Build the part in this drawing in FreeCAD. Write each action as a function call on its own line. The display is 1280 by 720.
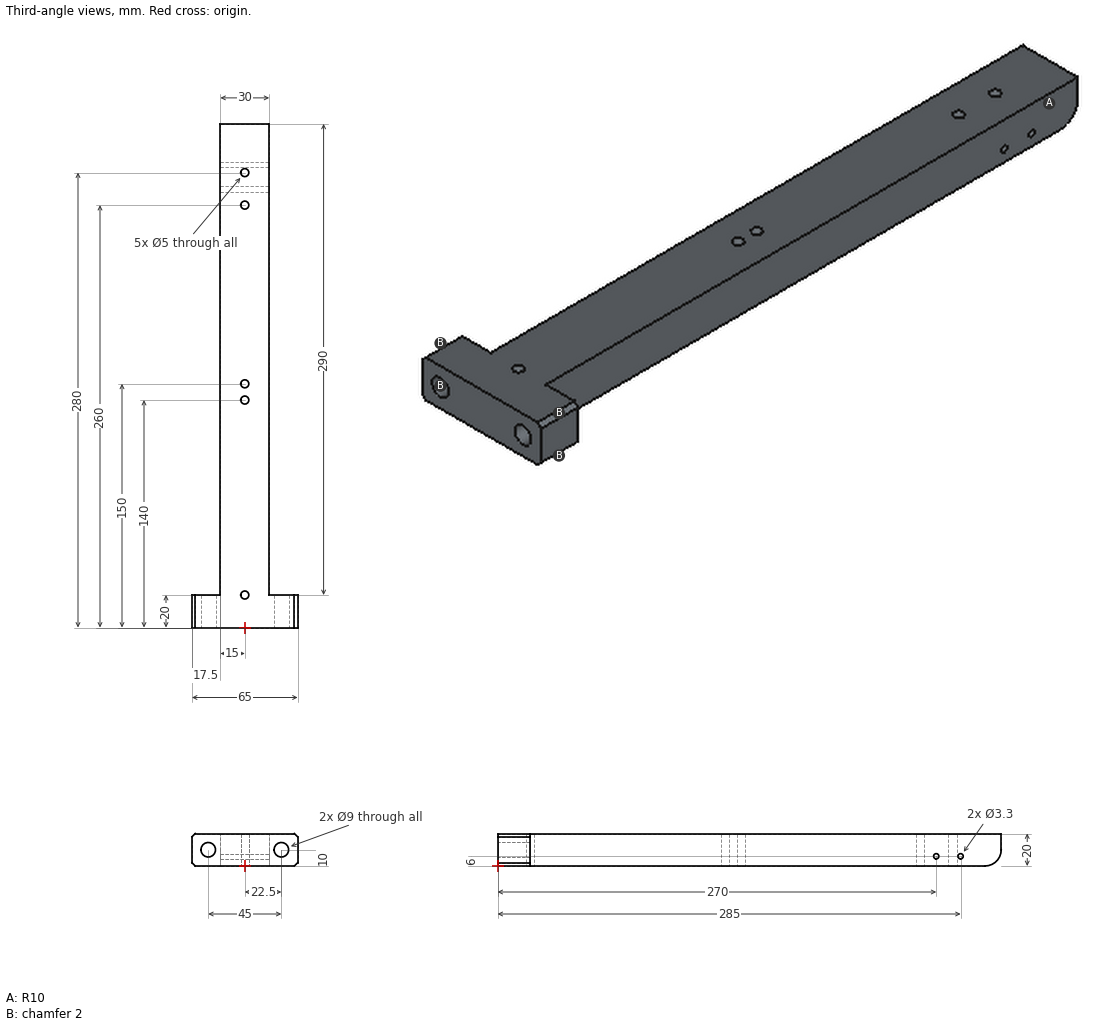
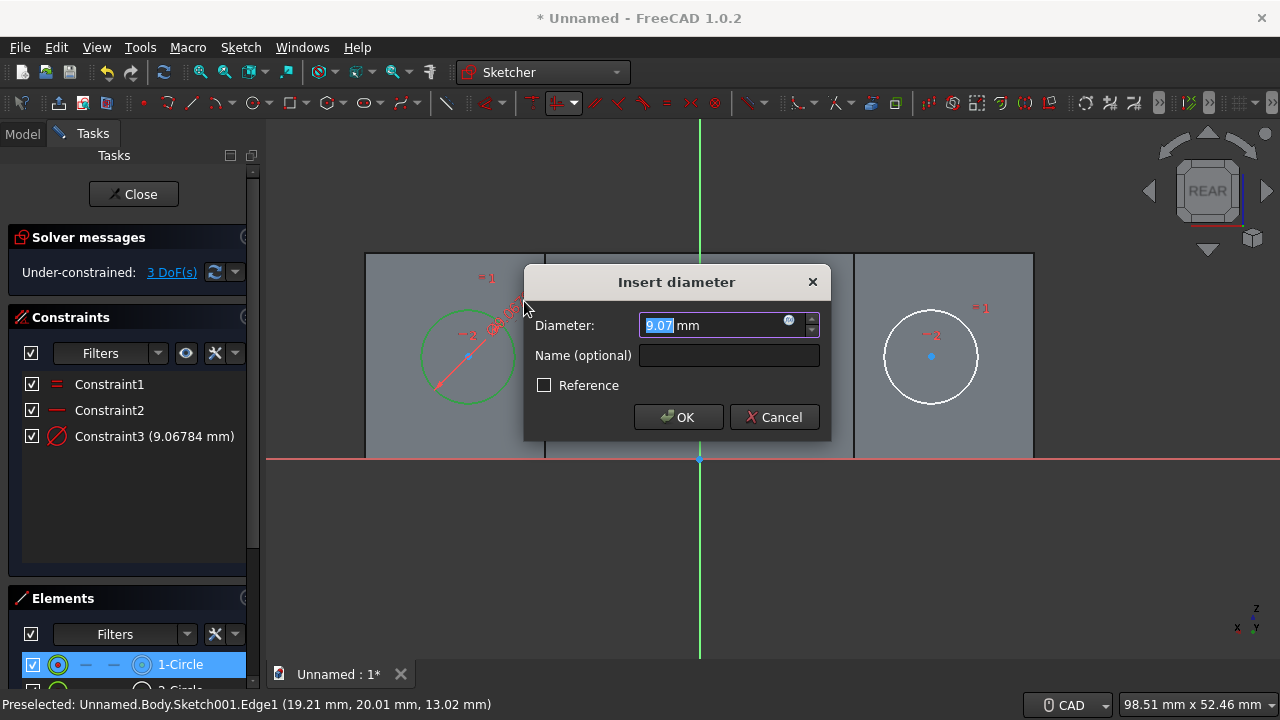
text(9)
key(Return)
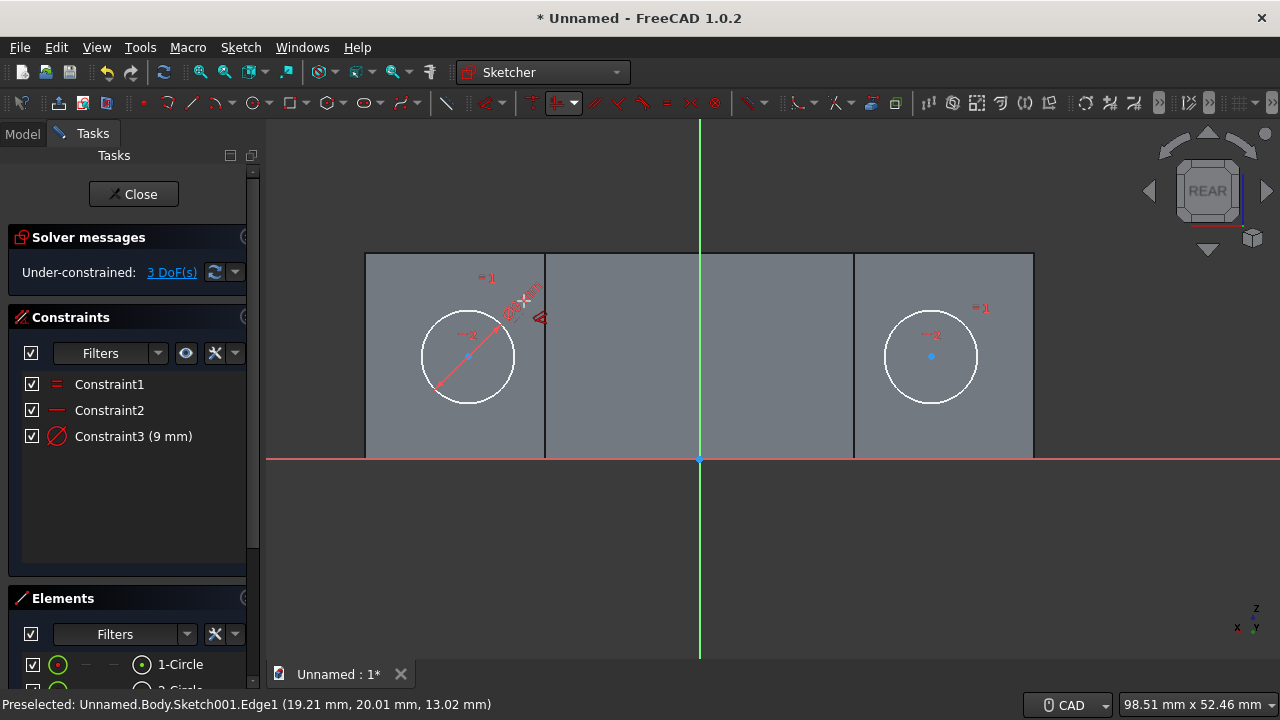
click(468, 357)
click(434, 408)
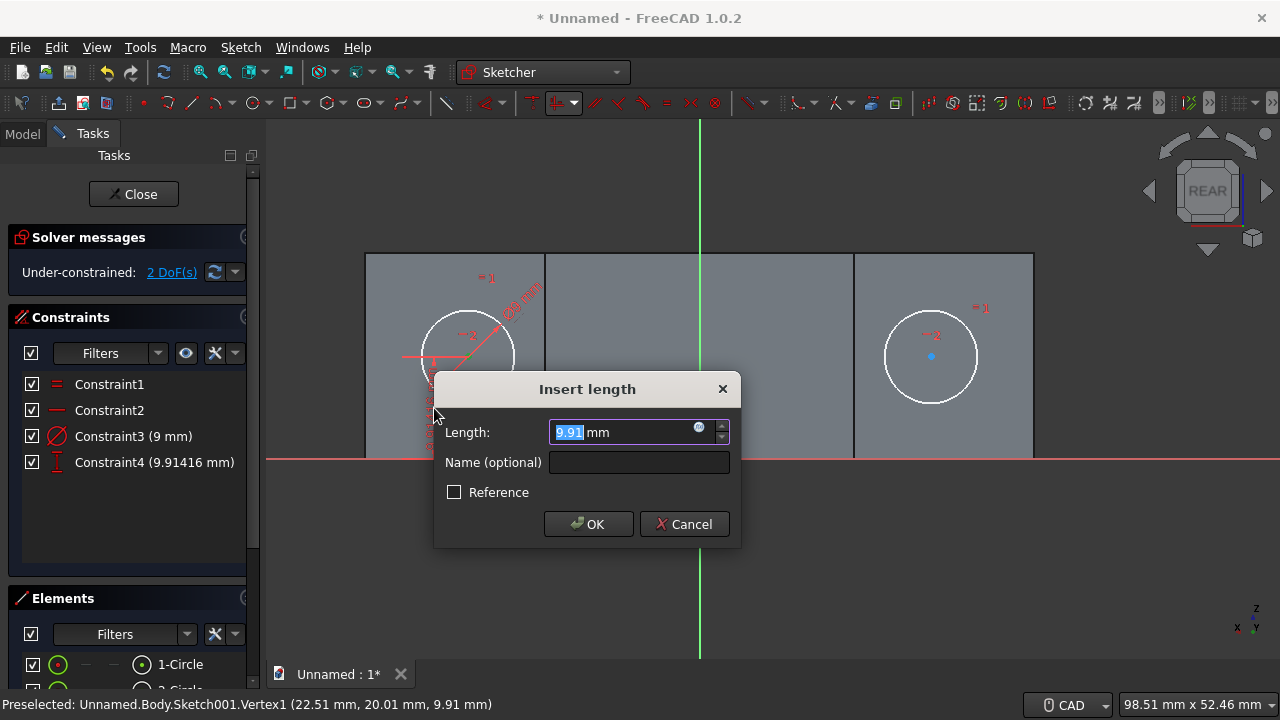
text(10)
key(Return)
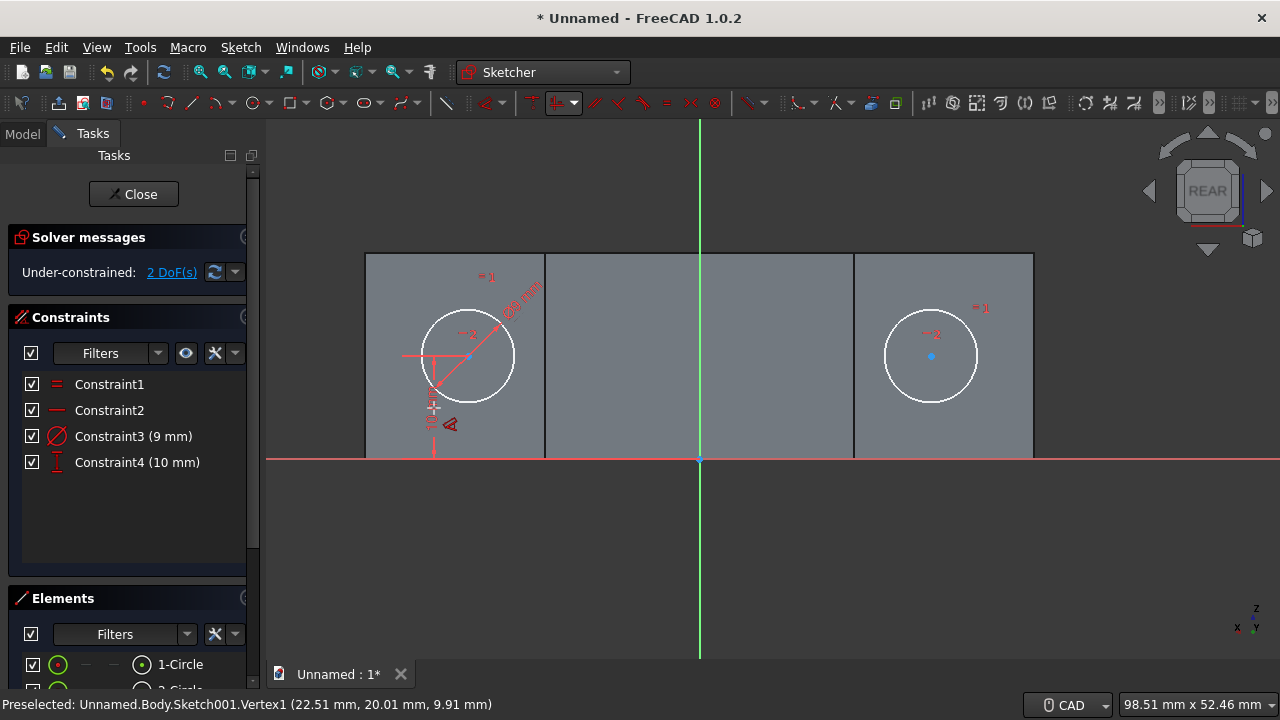
click(468, 356)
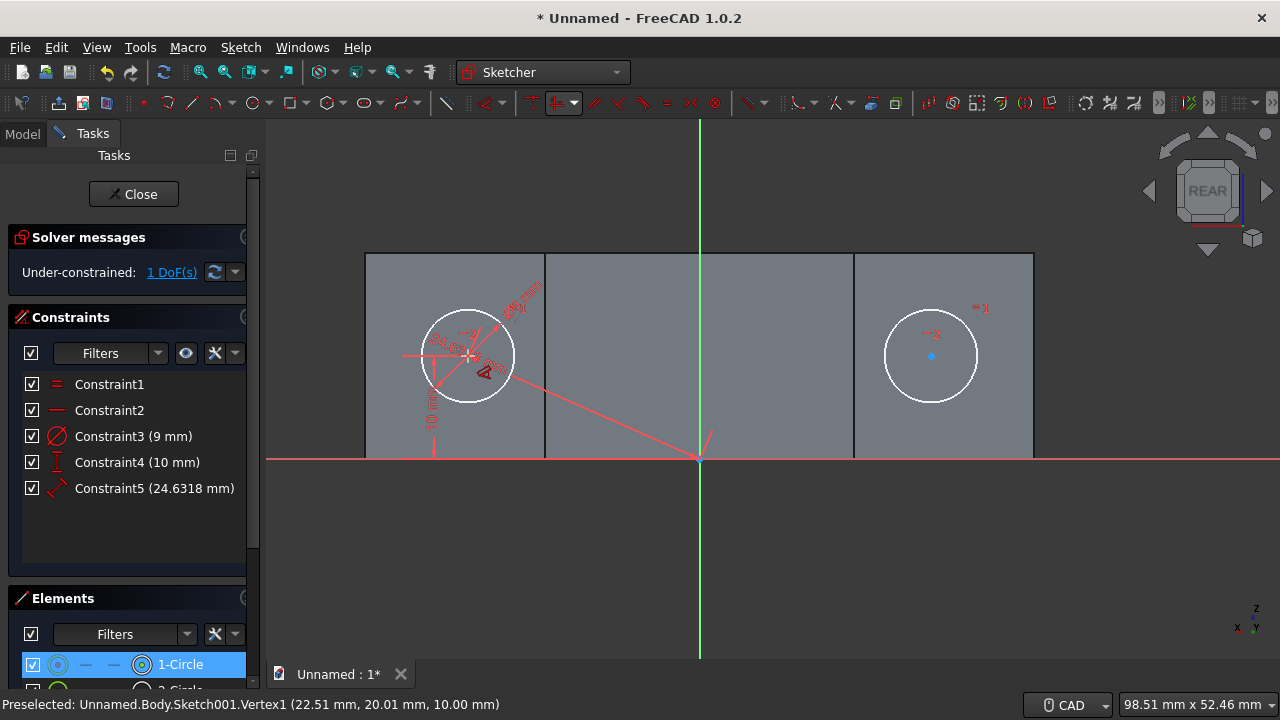
click(931, 356)
click(593, 322)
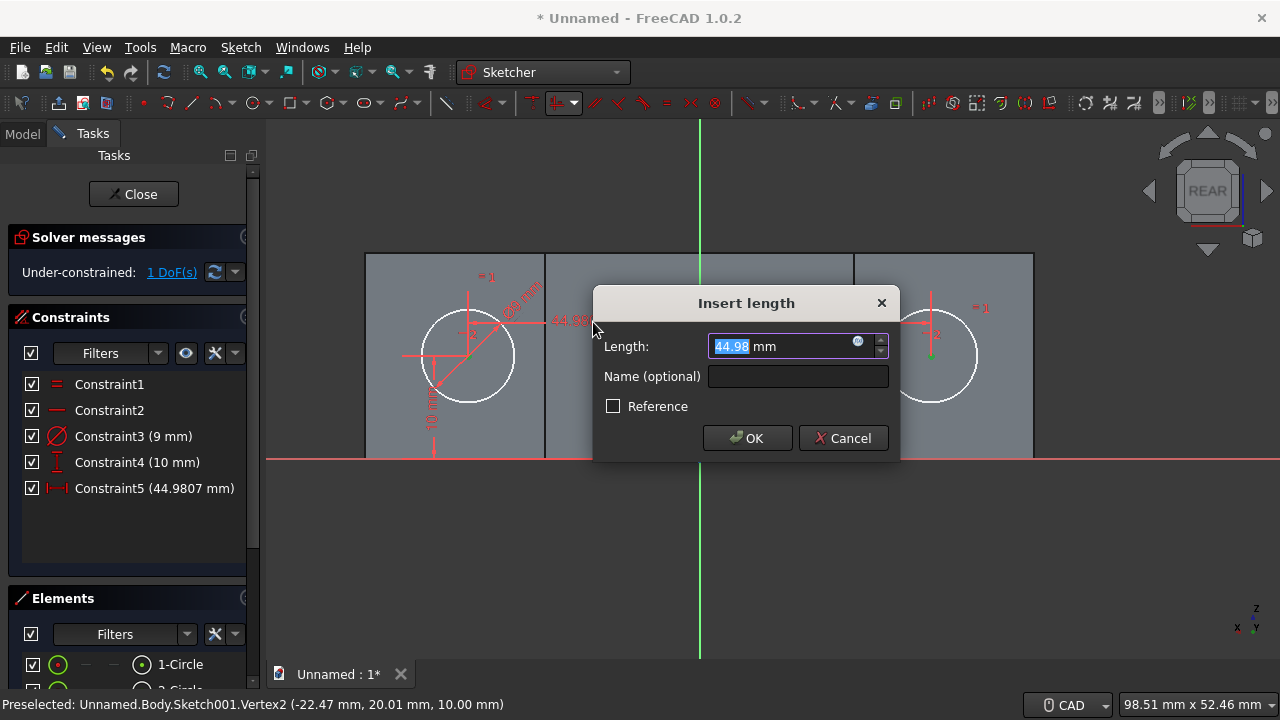
text(45)
key(Return)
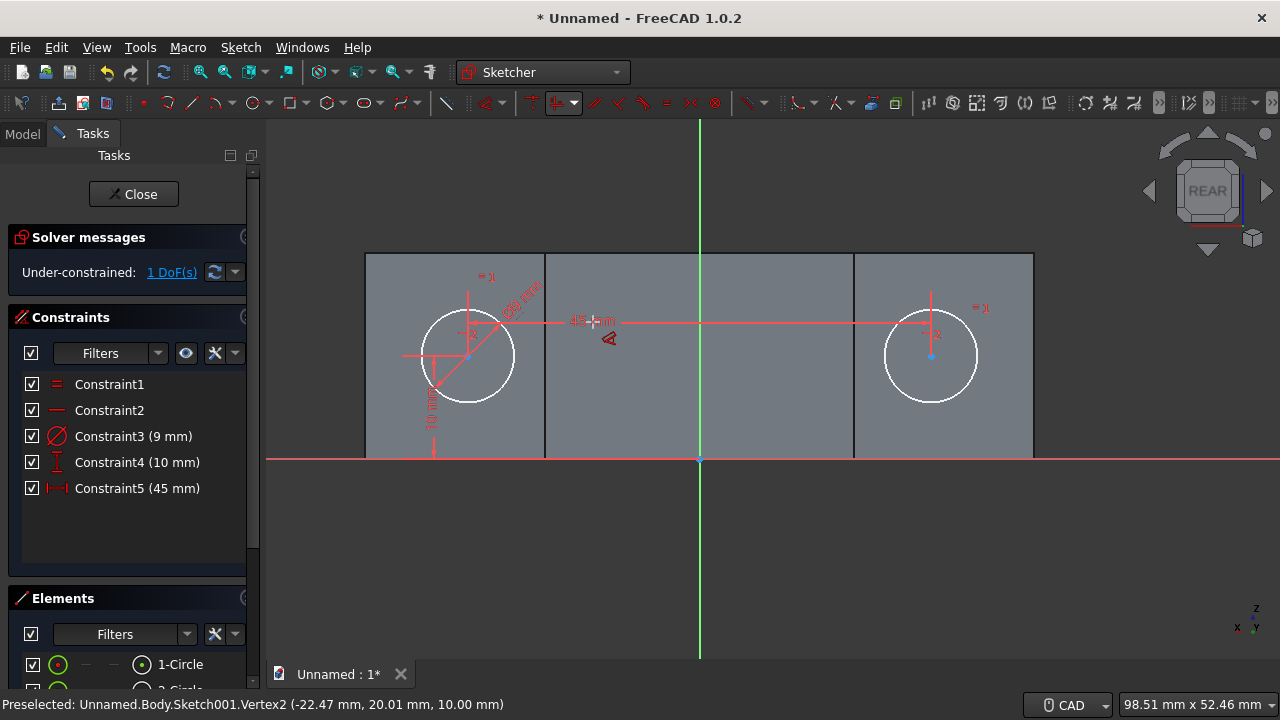
click(468, 356)
click(584, 493)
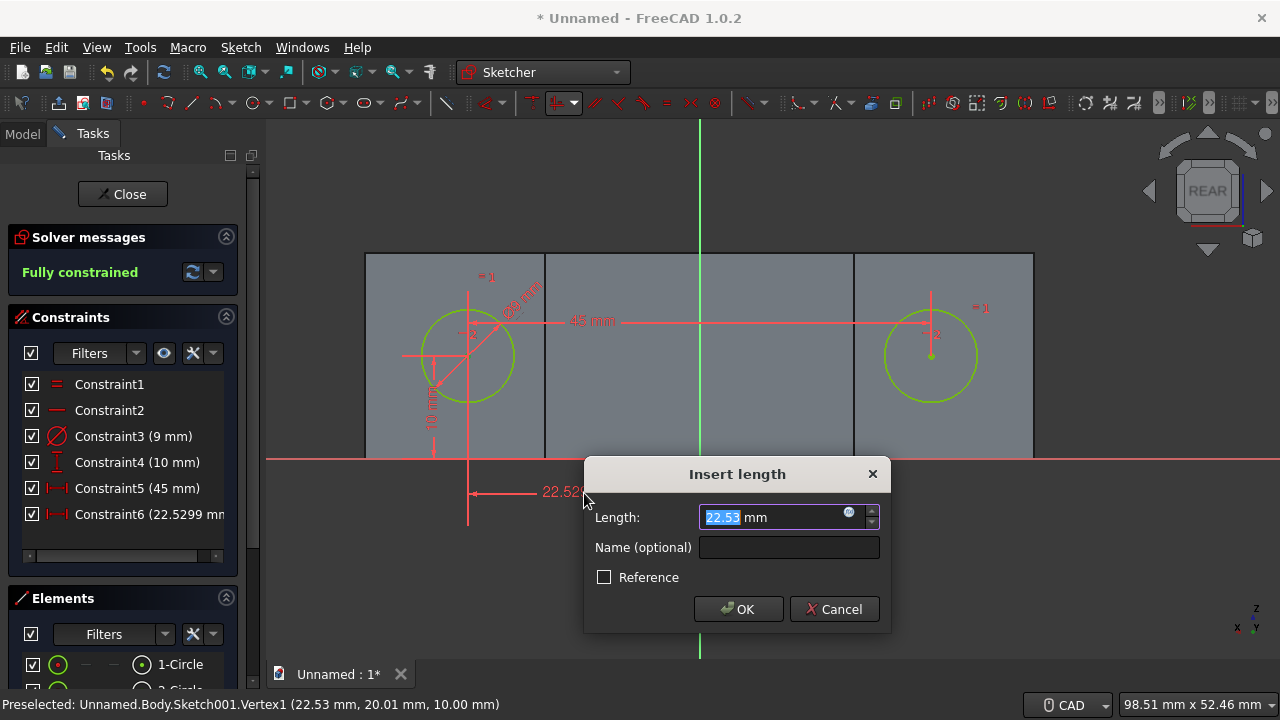
text(22.5)
key(Return)
key(Escape)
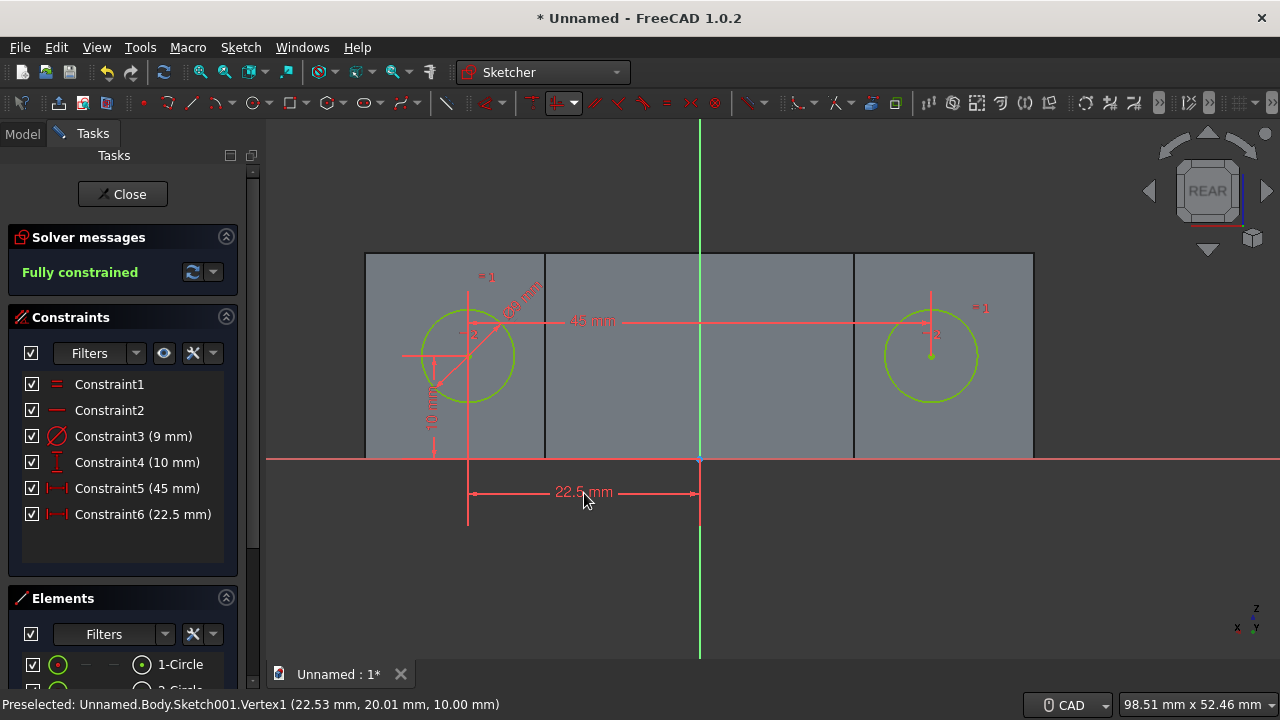
click(123, 194)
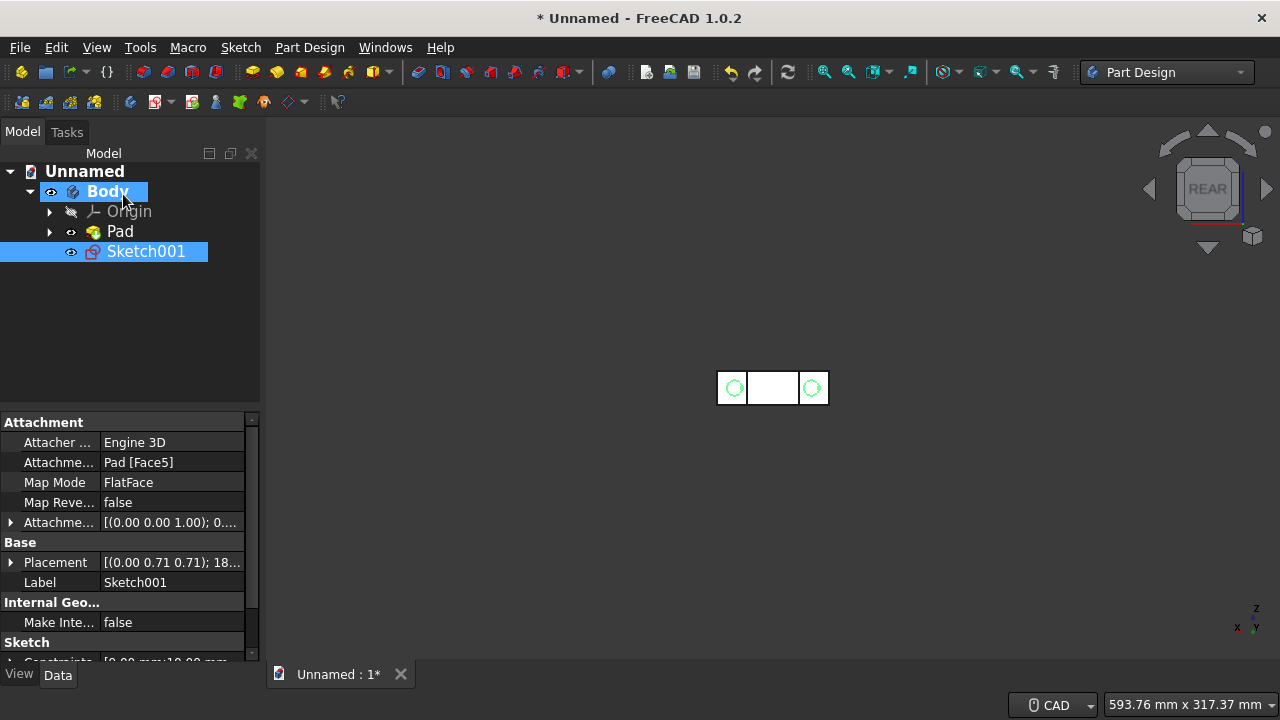
click(444, 72)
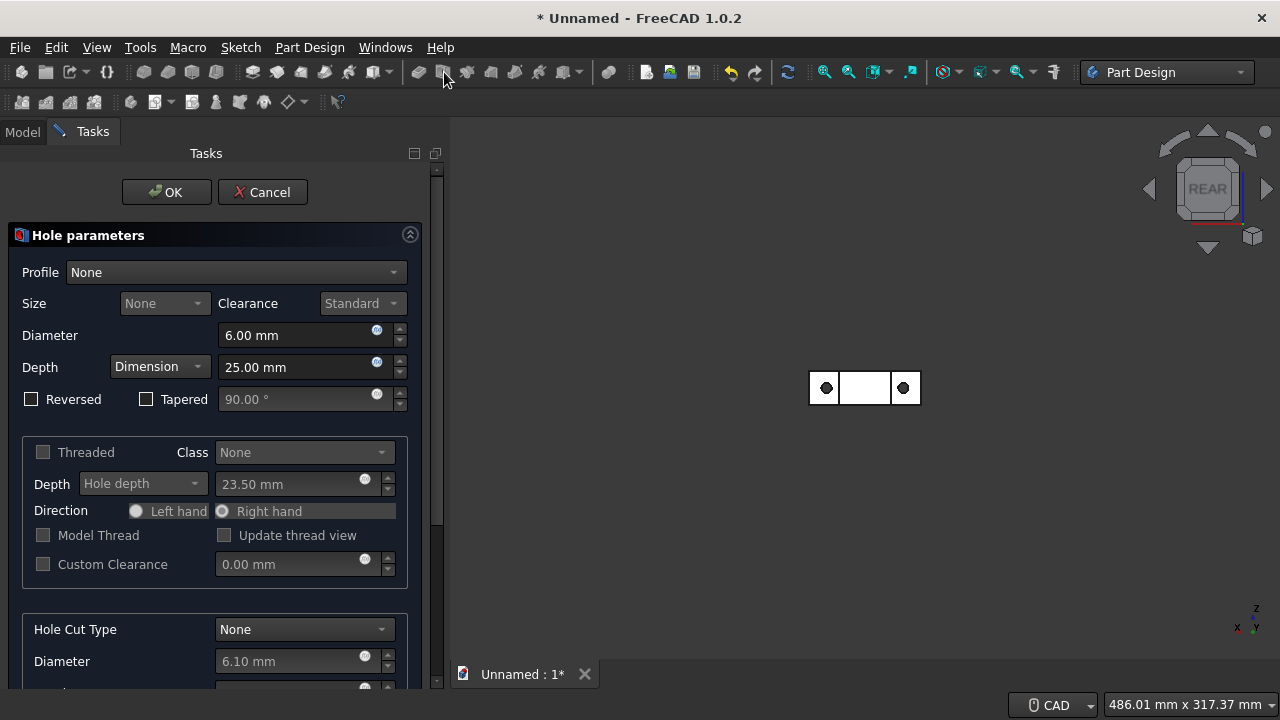
triple_click(305, 335)